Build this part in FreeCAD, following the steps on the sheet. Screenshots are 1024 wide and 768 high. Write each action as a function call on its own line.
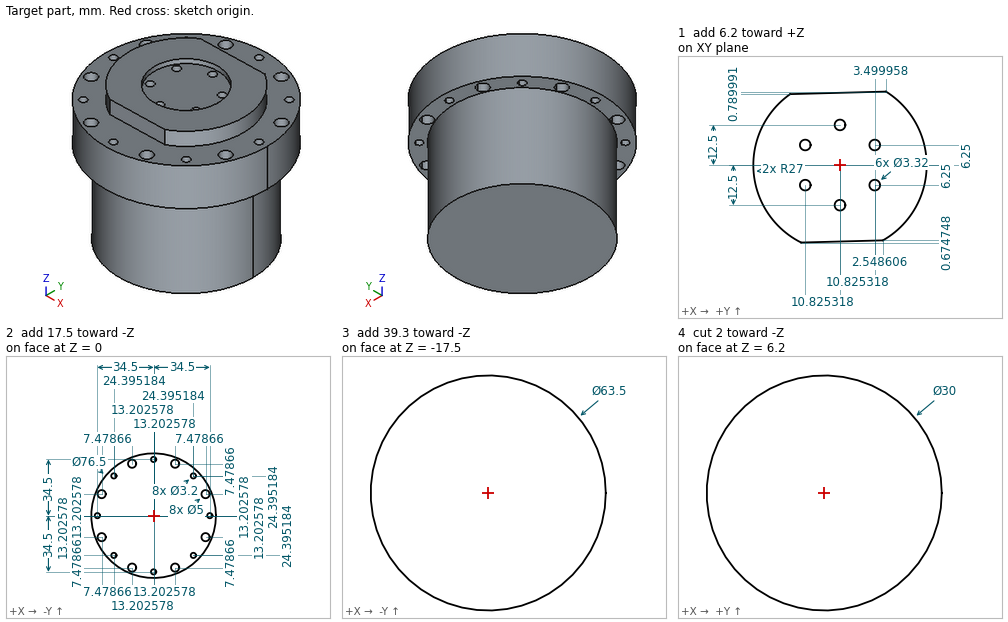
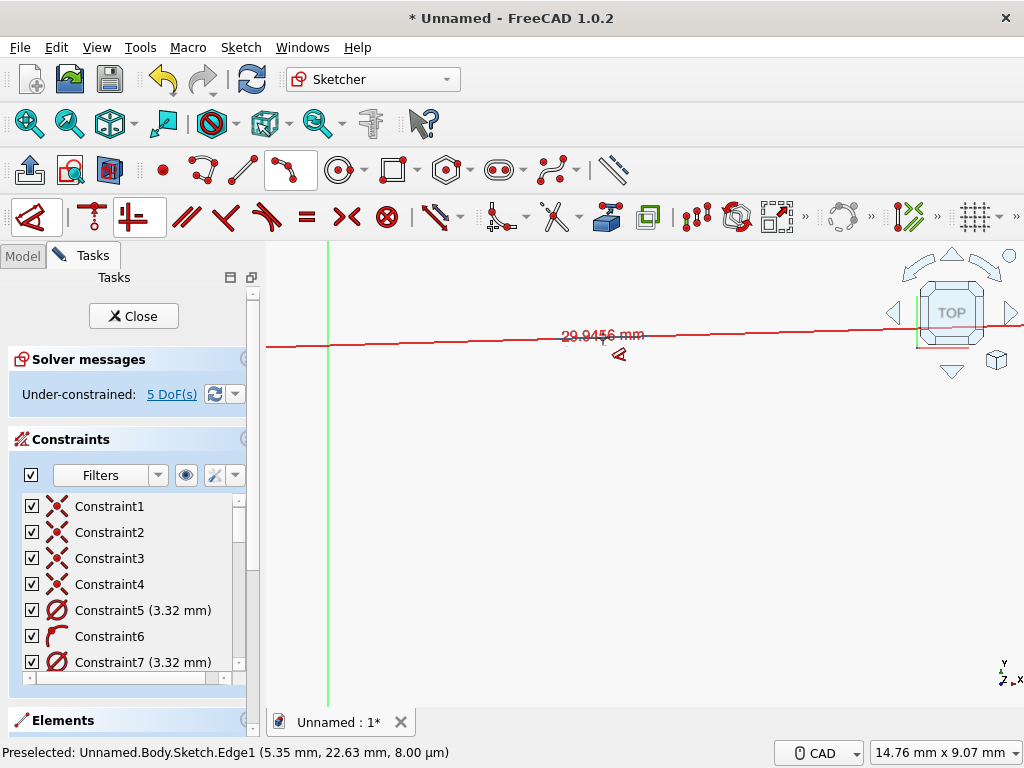
key(Escape)
key(Escape)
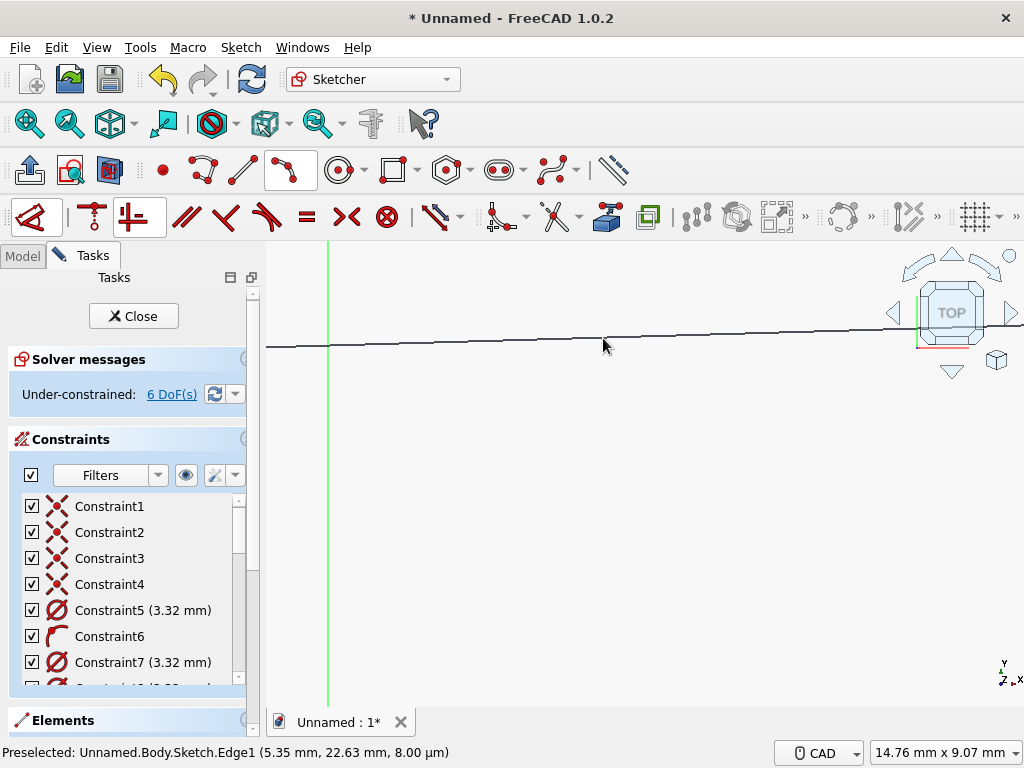
click(603, 338)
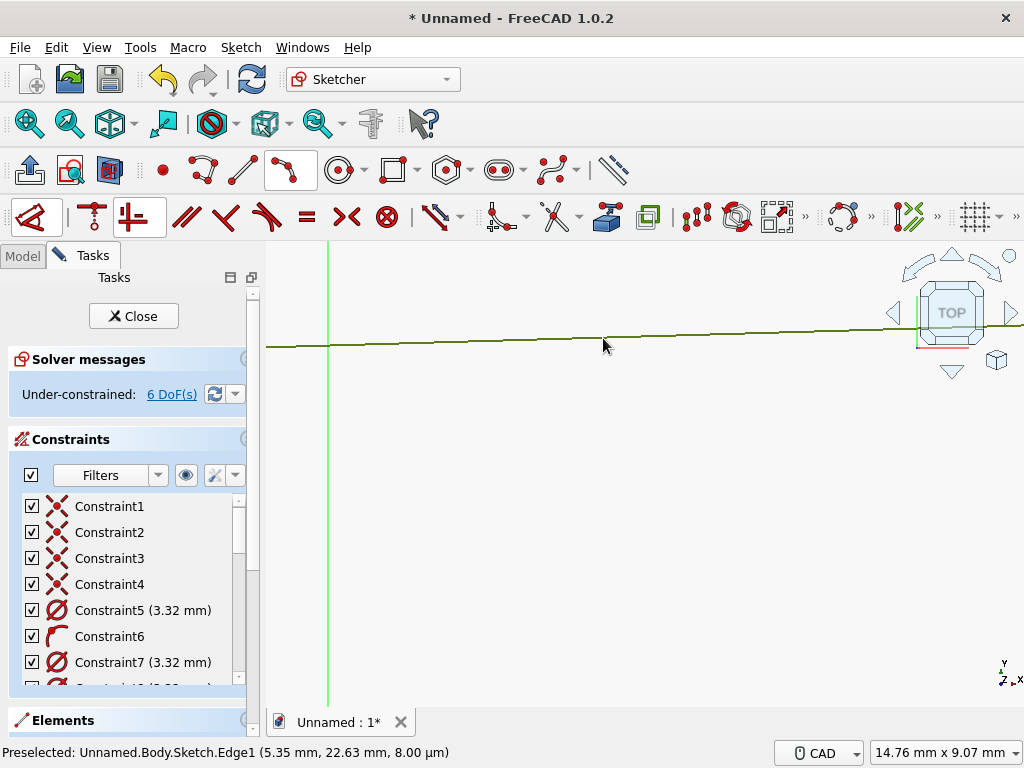
key(i)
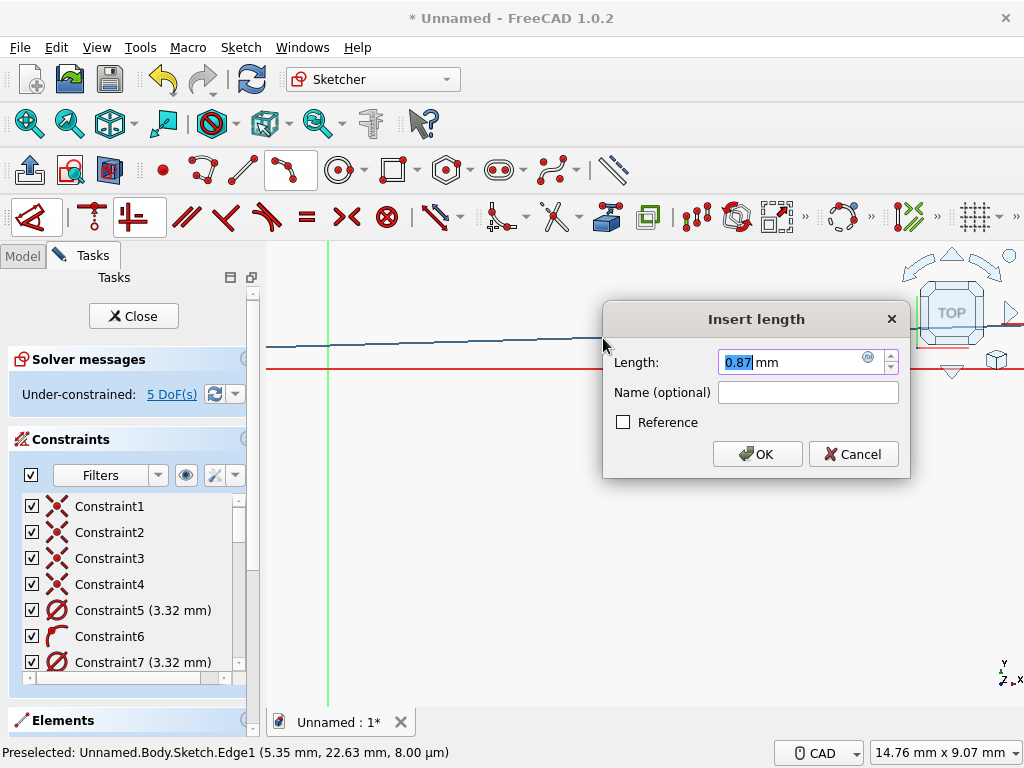
text(0.789991)
key(Return)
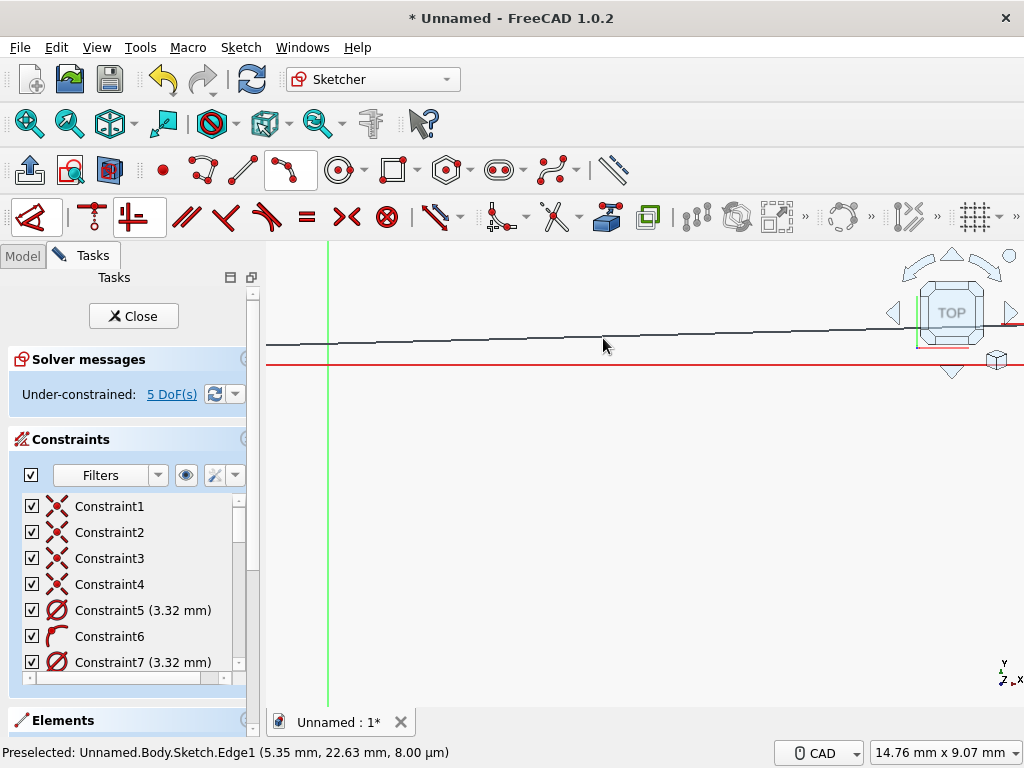
scroll(607, 342, down, 11)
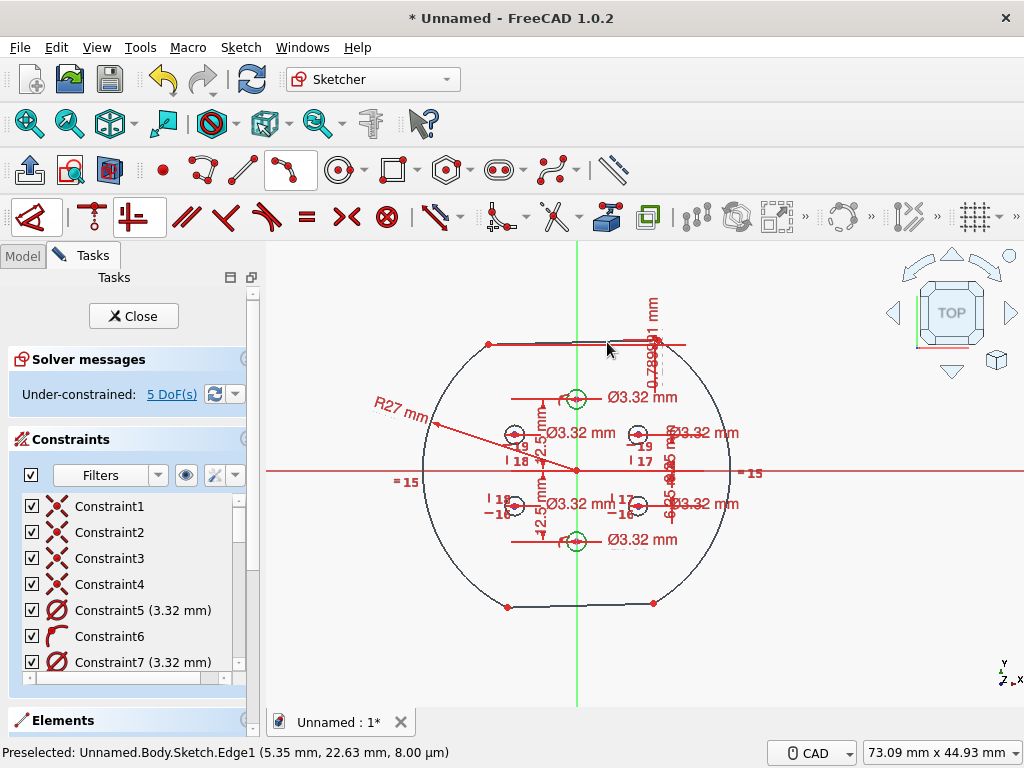
scroll(551, 606, up, 12)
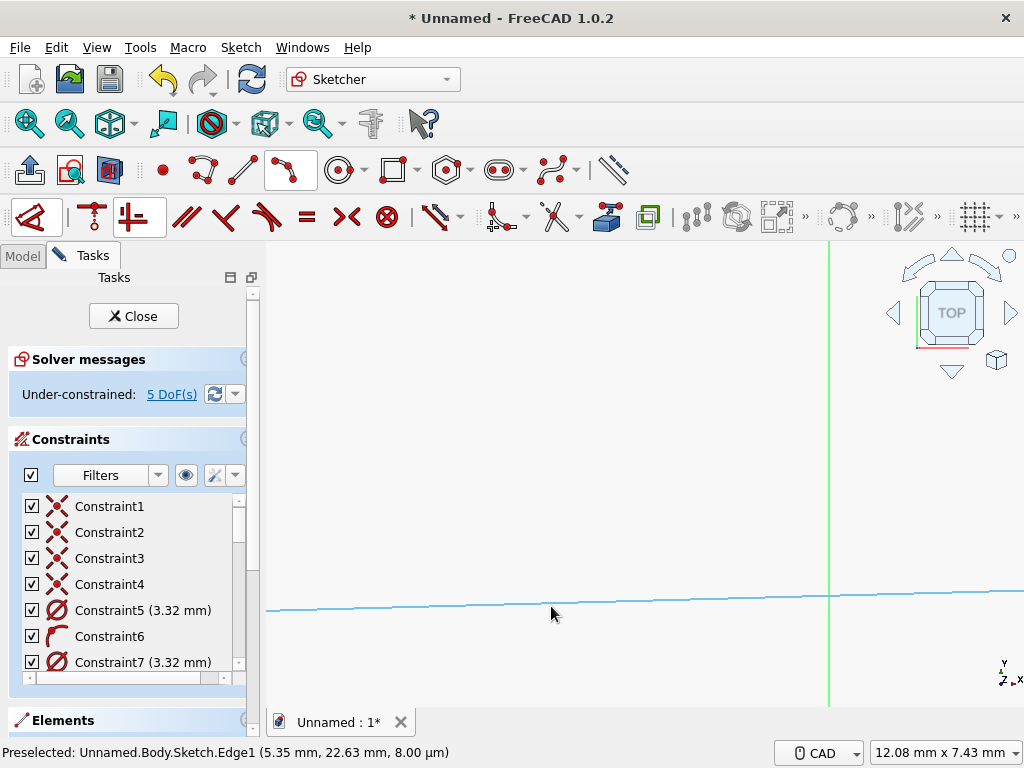
click(547, 603)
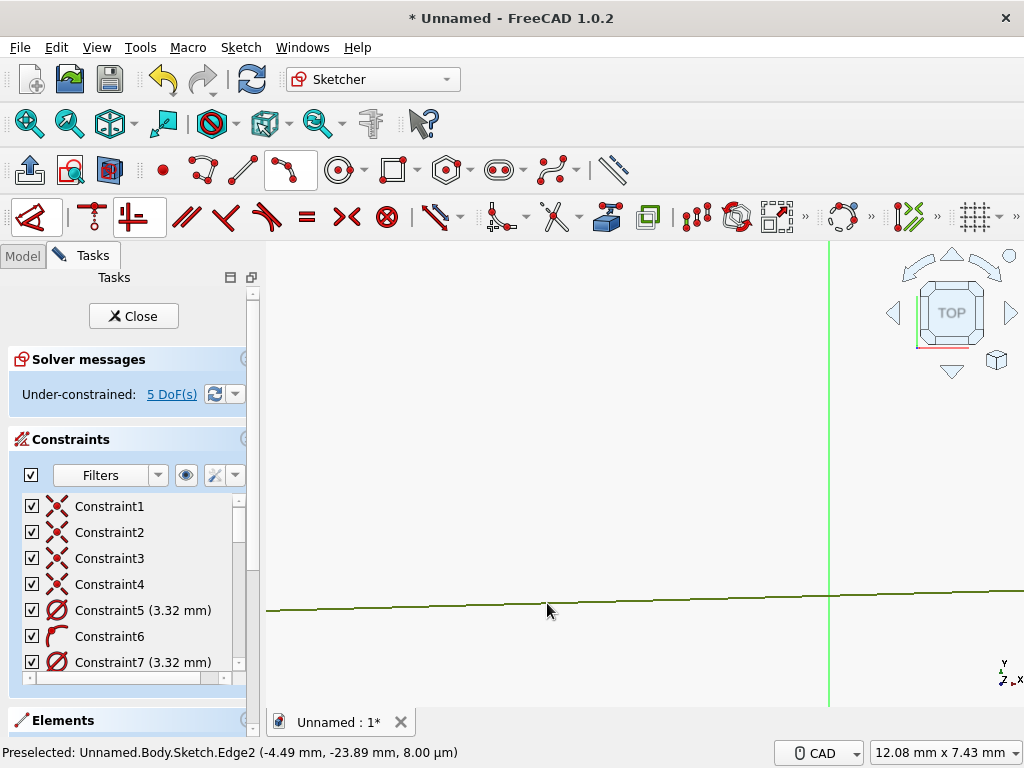
click(56, 218)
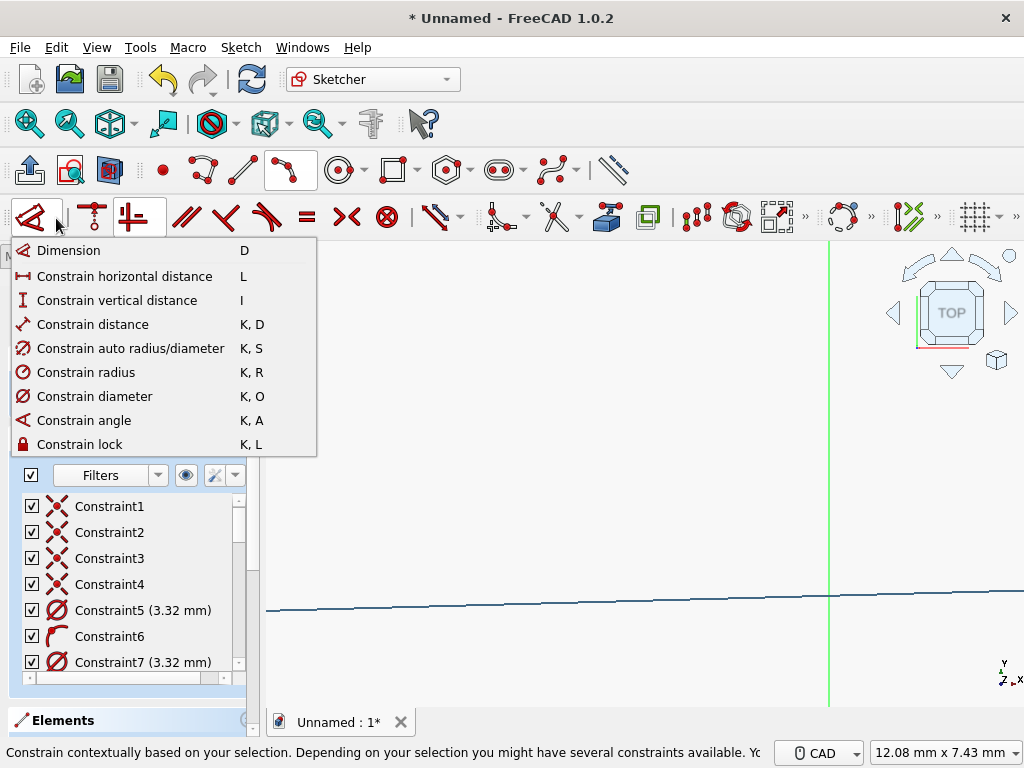
click(164, 300)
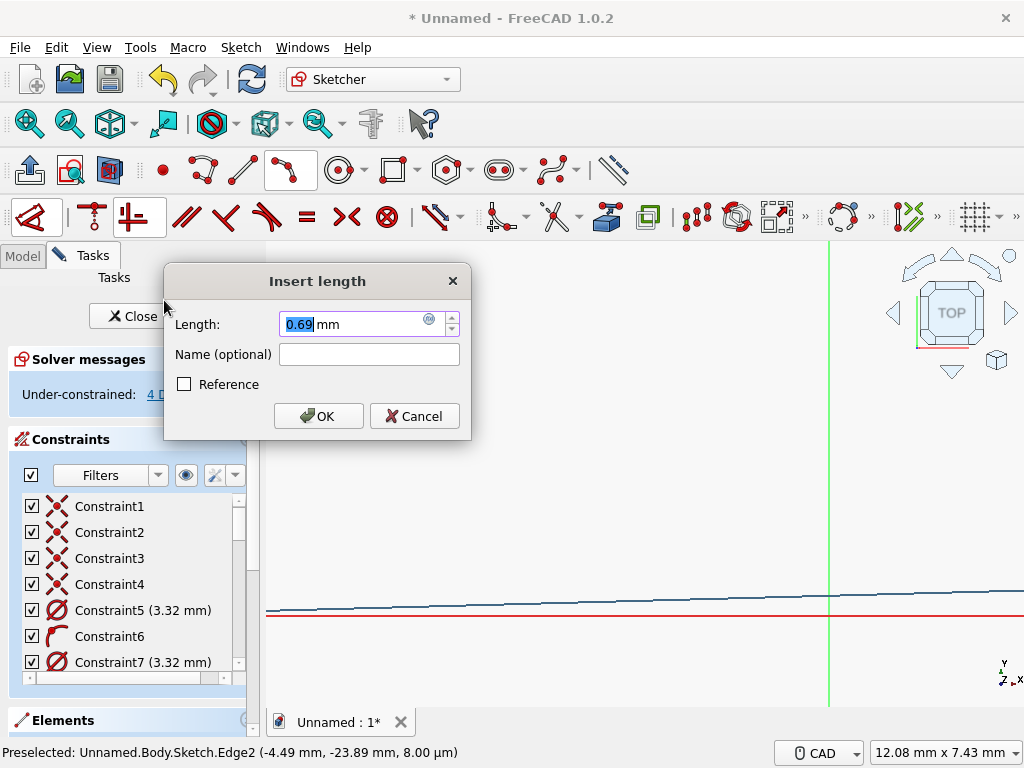
text(0.674748)
key(Return)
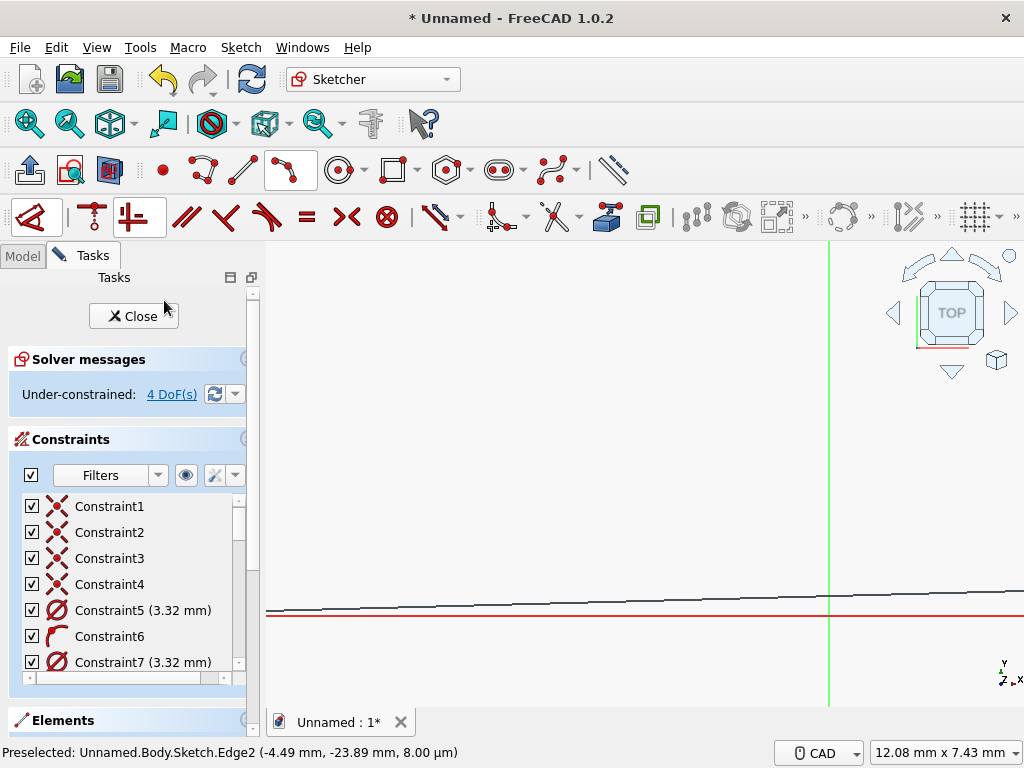
scroll(551, 607, down, 12)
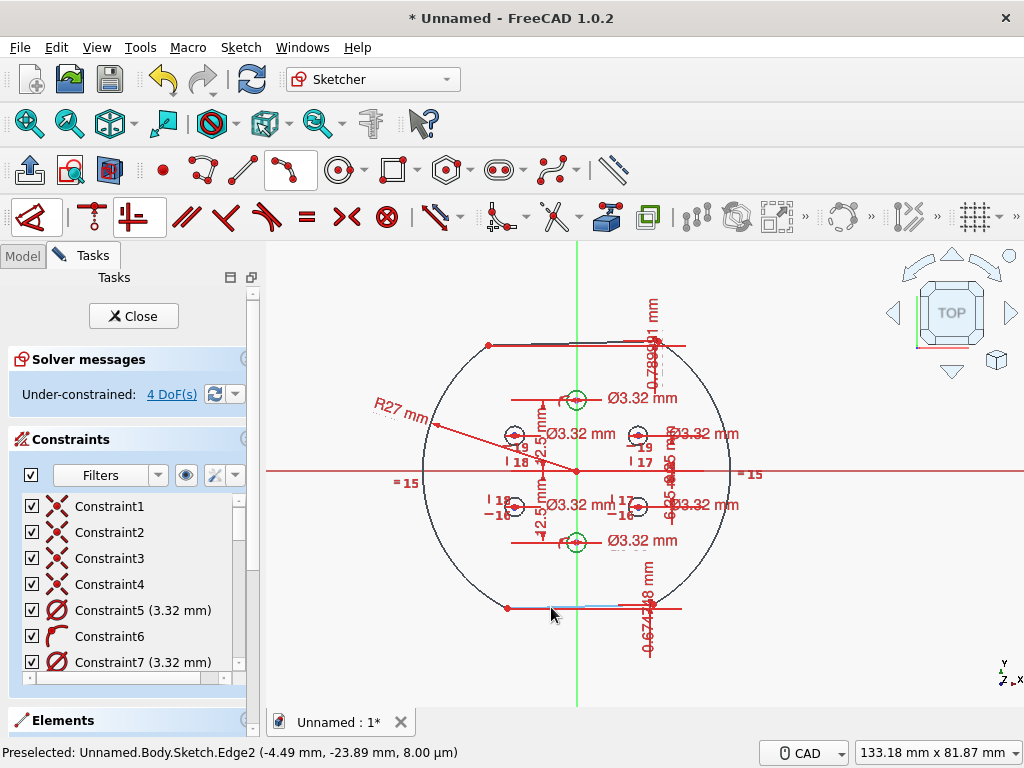
click(638, 507)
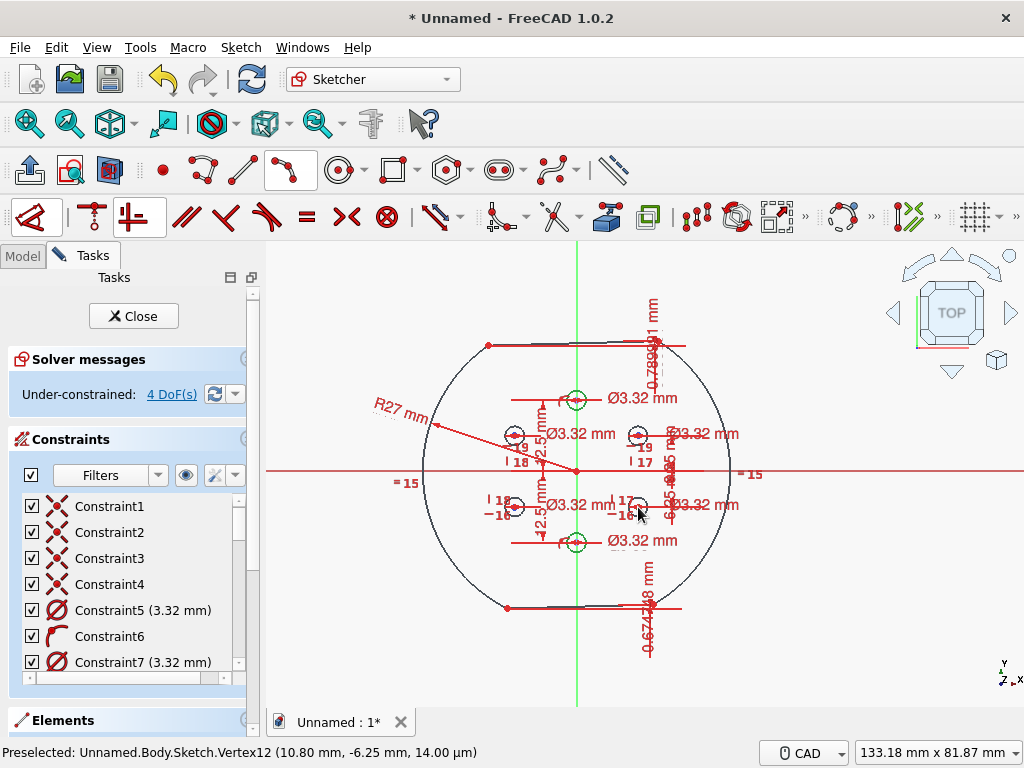
key(l)